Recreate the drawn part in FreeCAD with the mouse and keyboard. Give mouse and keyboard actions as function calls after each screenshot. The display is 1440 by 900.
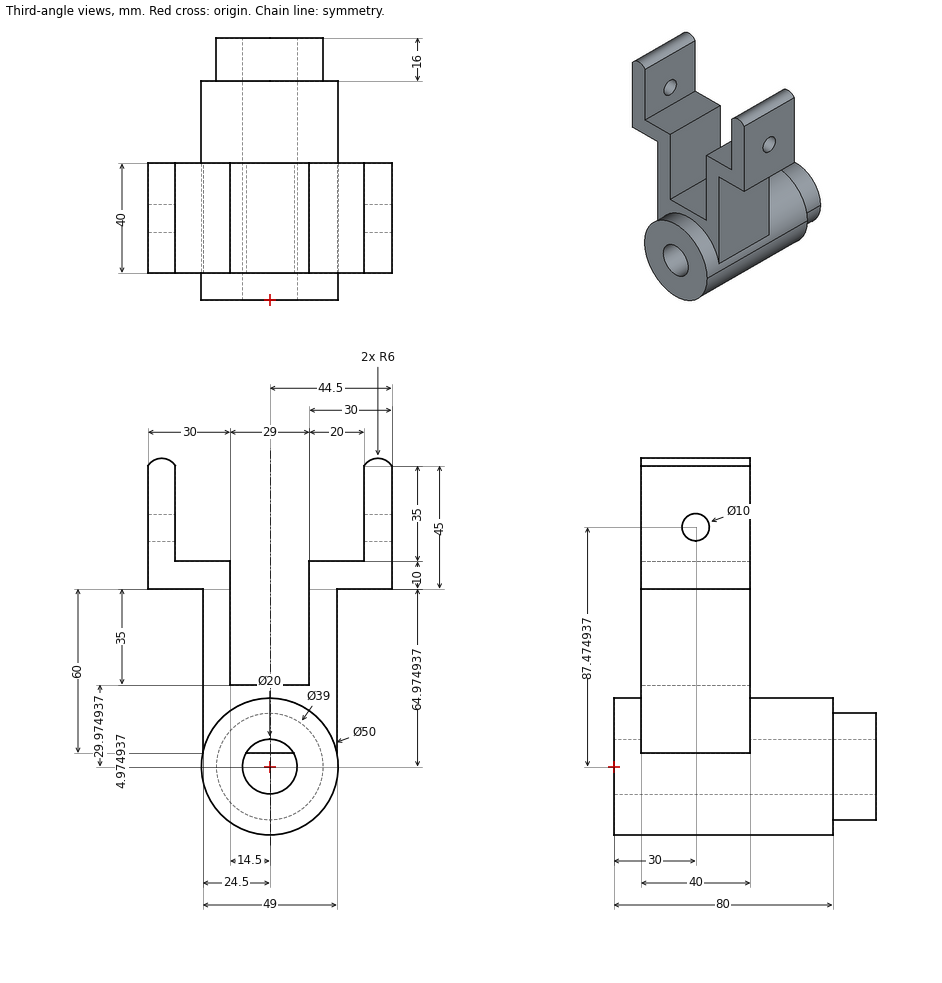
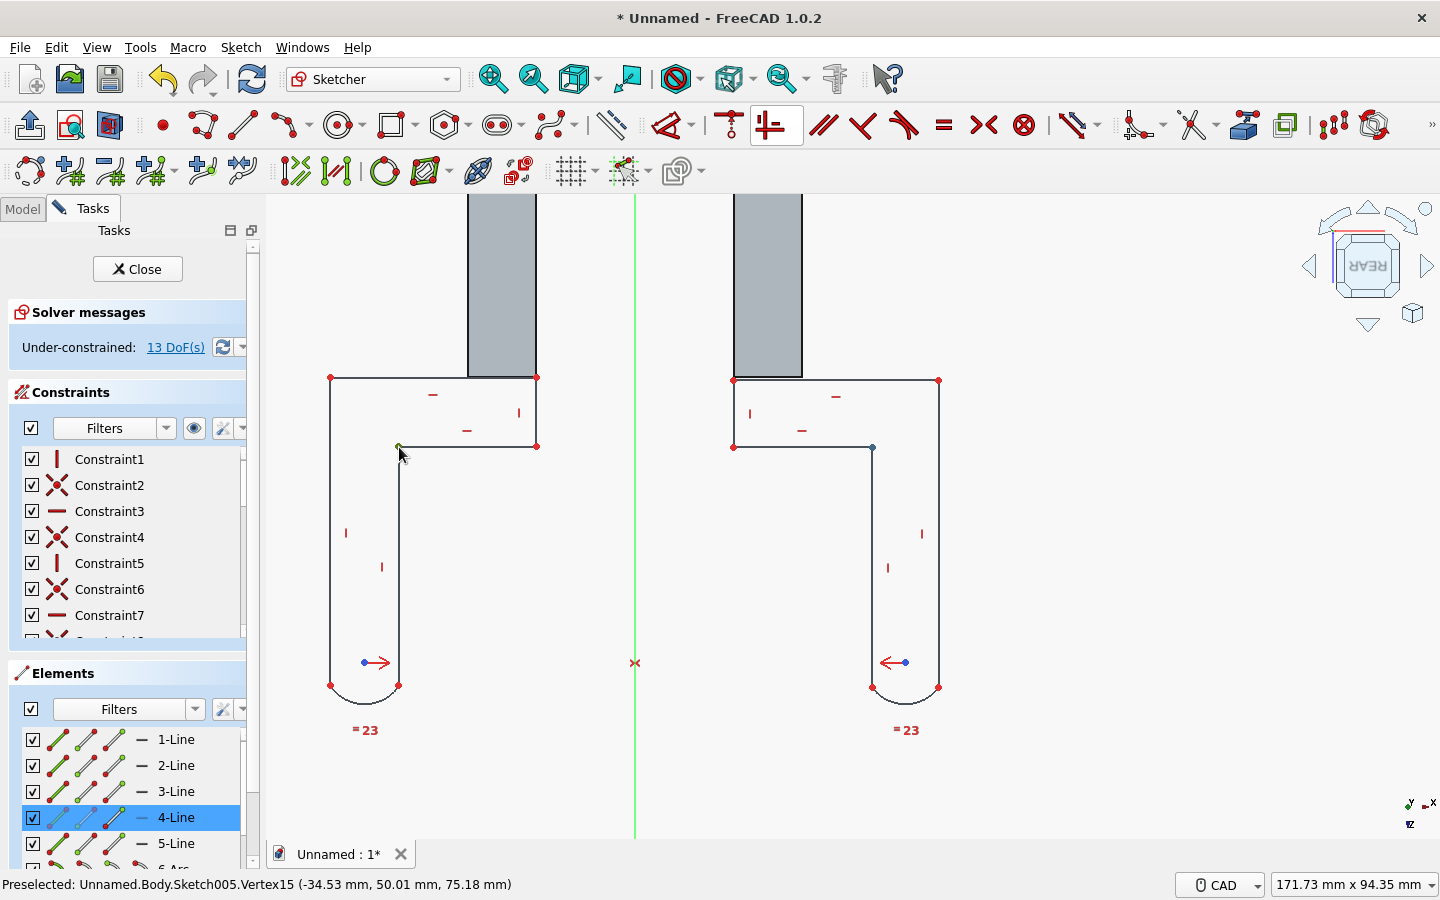
click(635, 769)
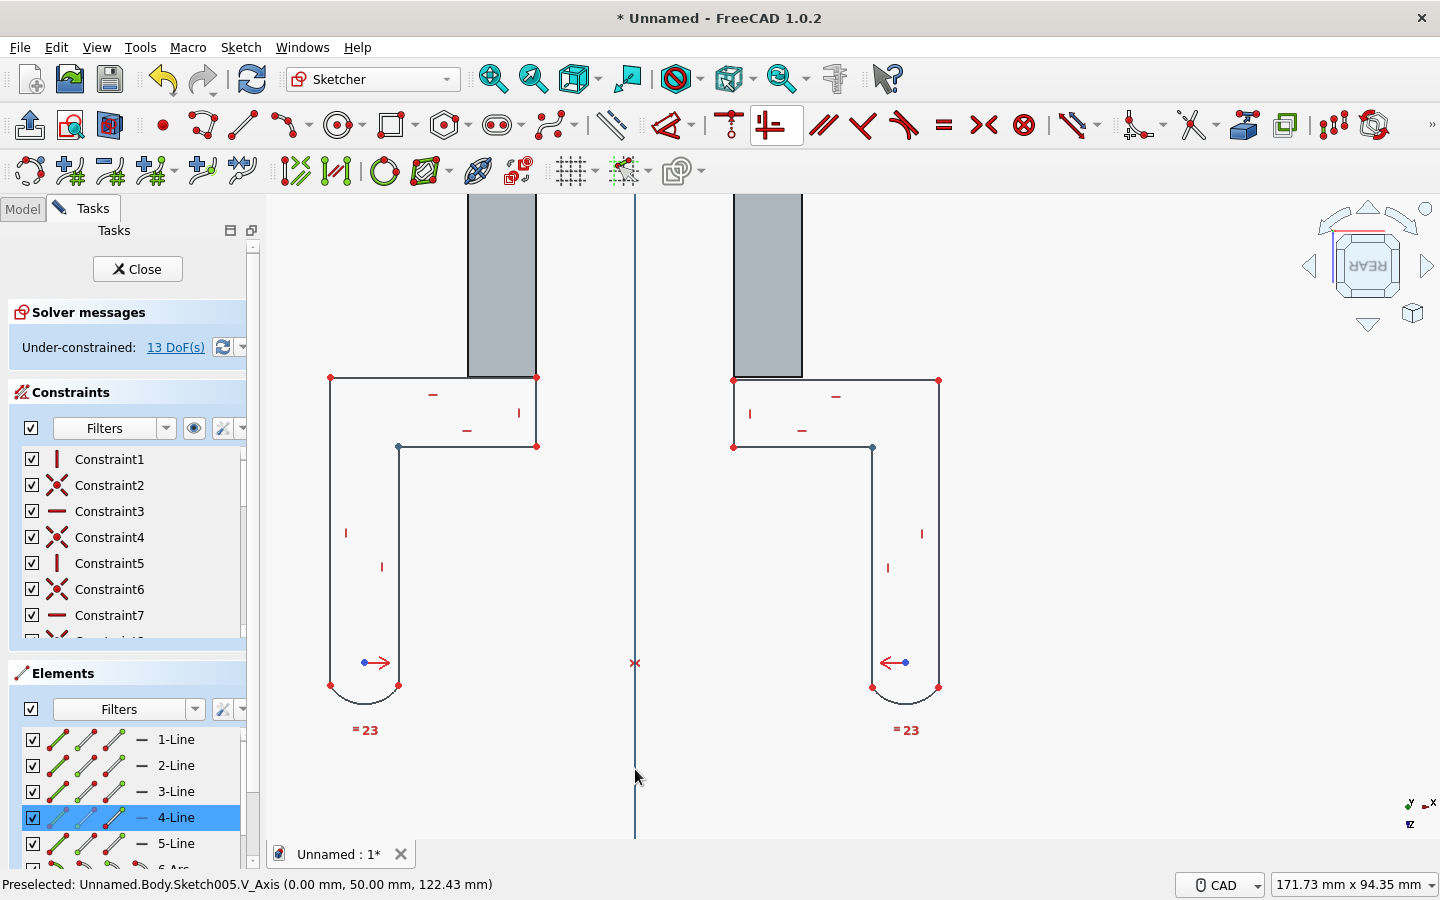
click(984, 126)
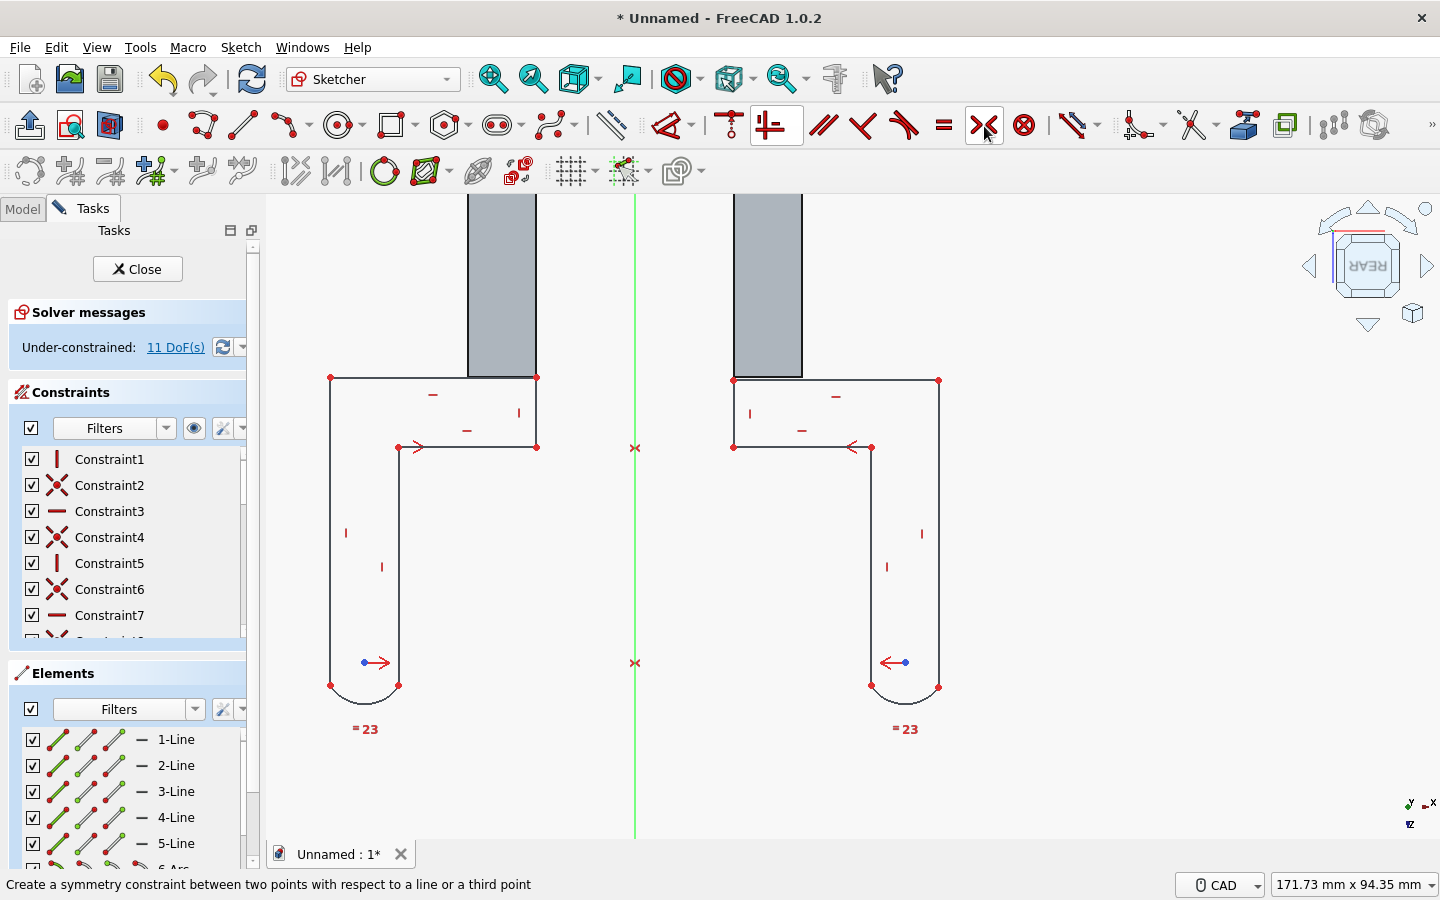
click(734, 380)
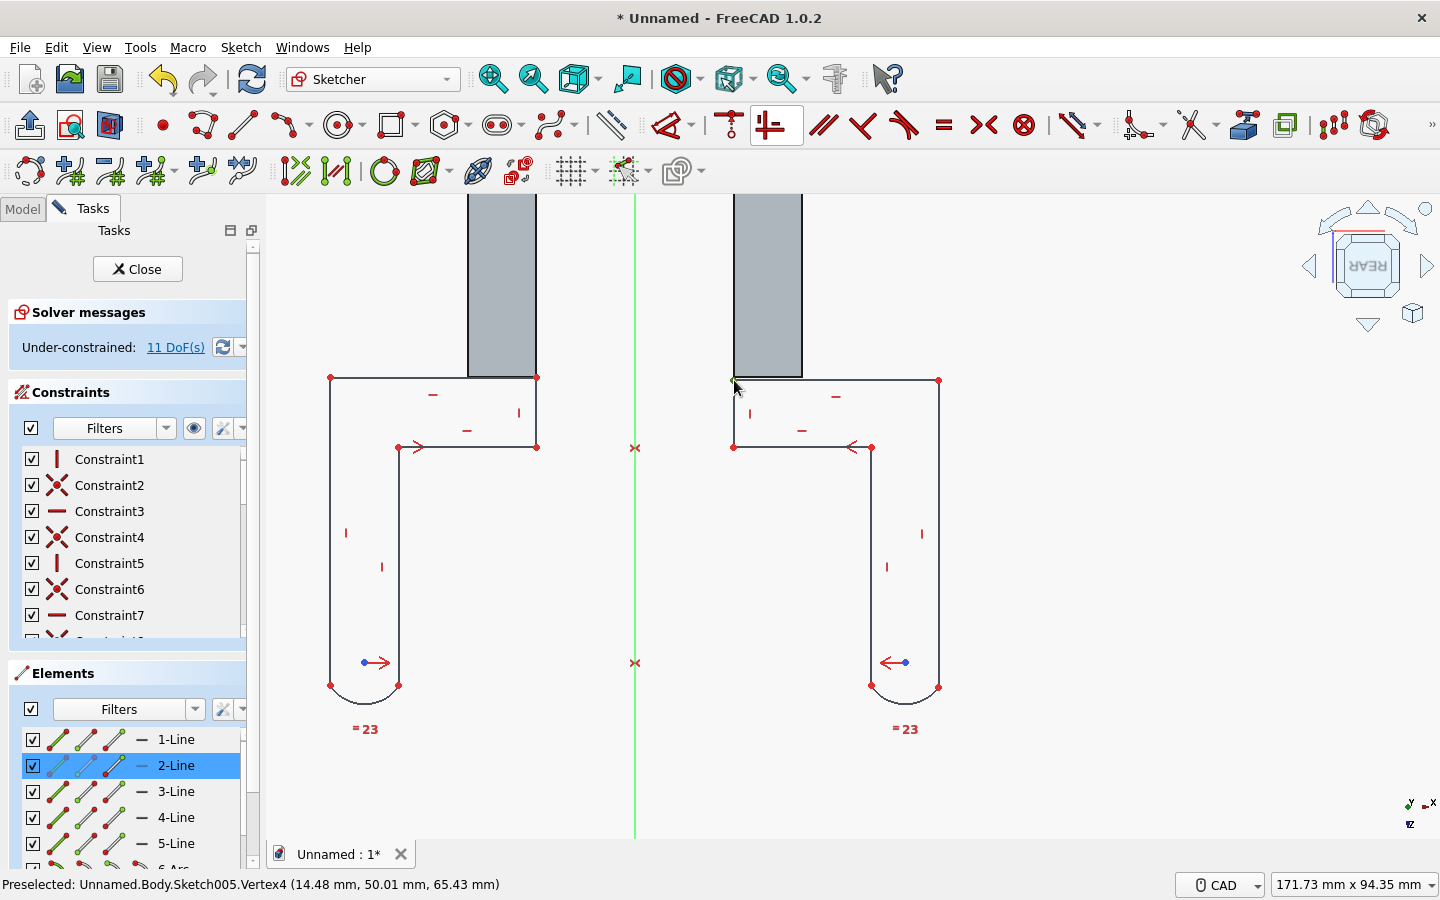
click(536, 378)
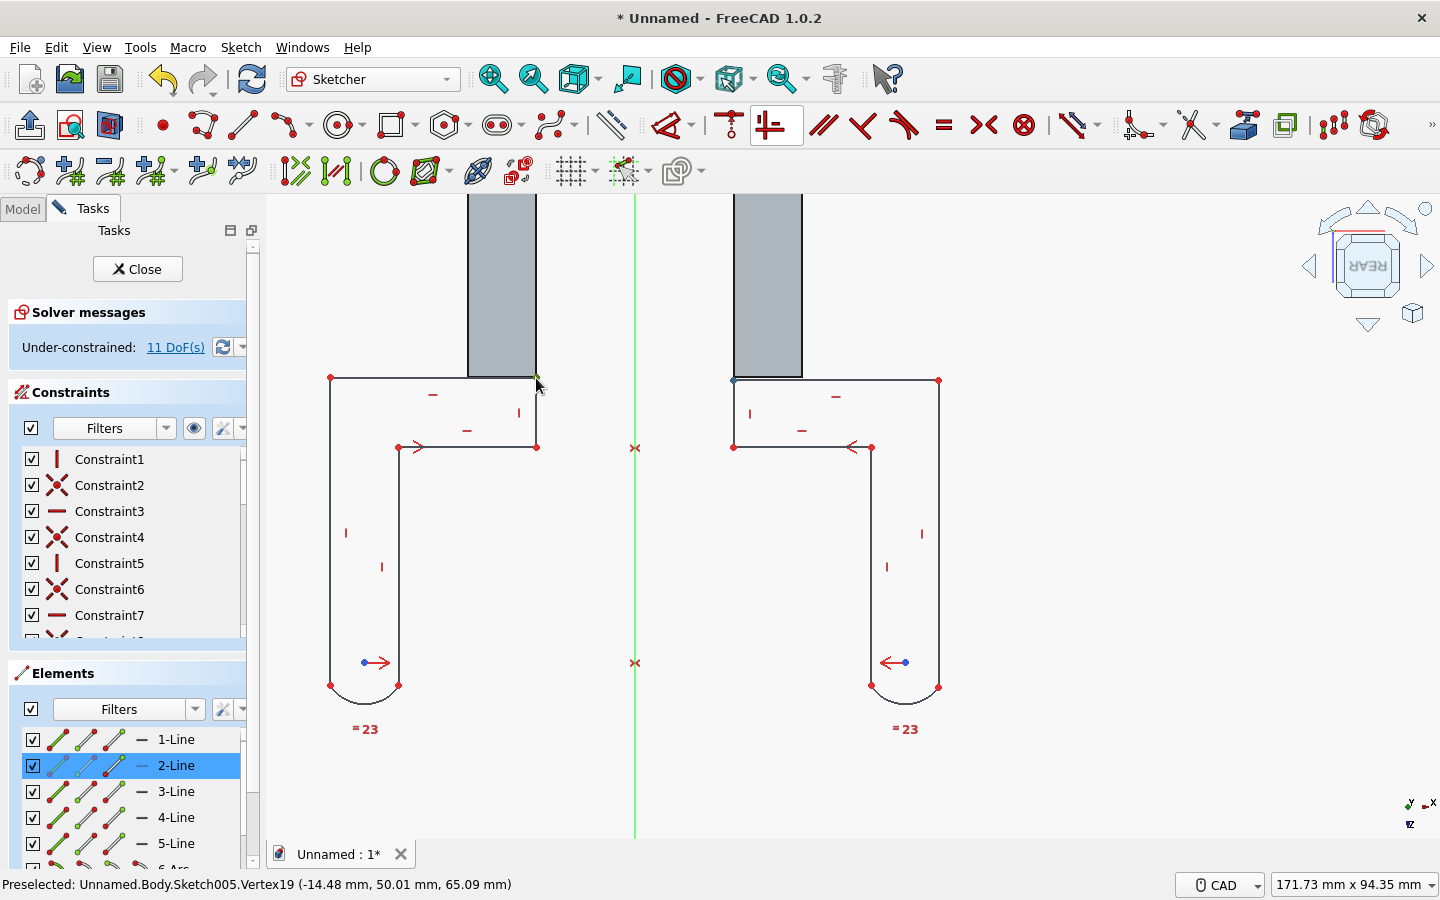
click(635, 769)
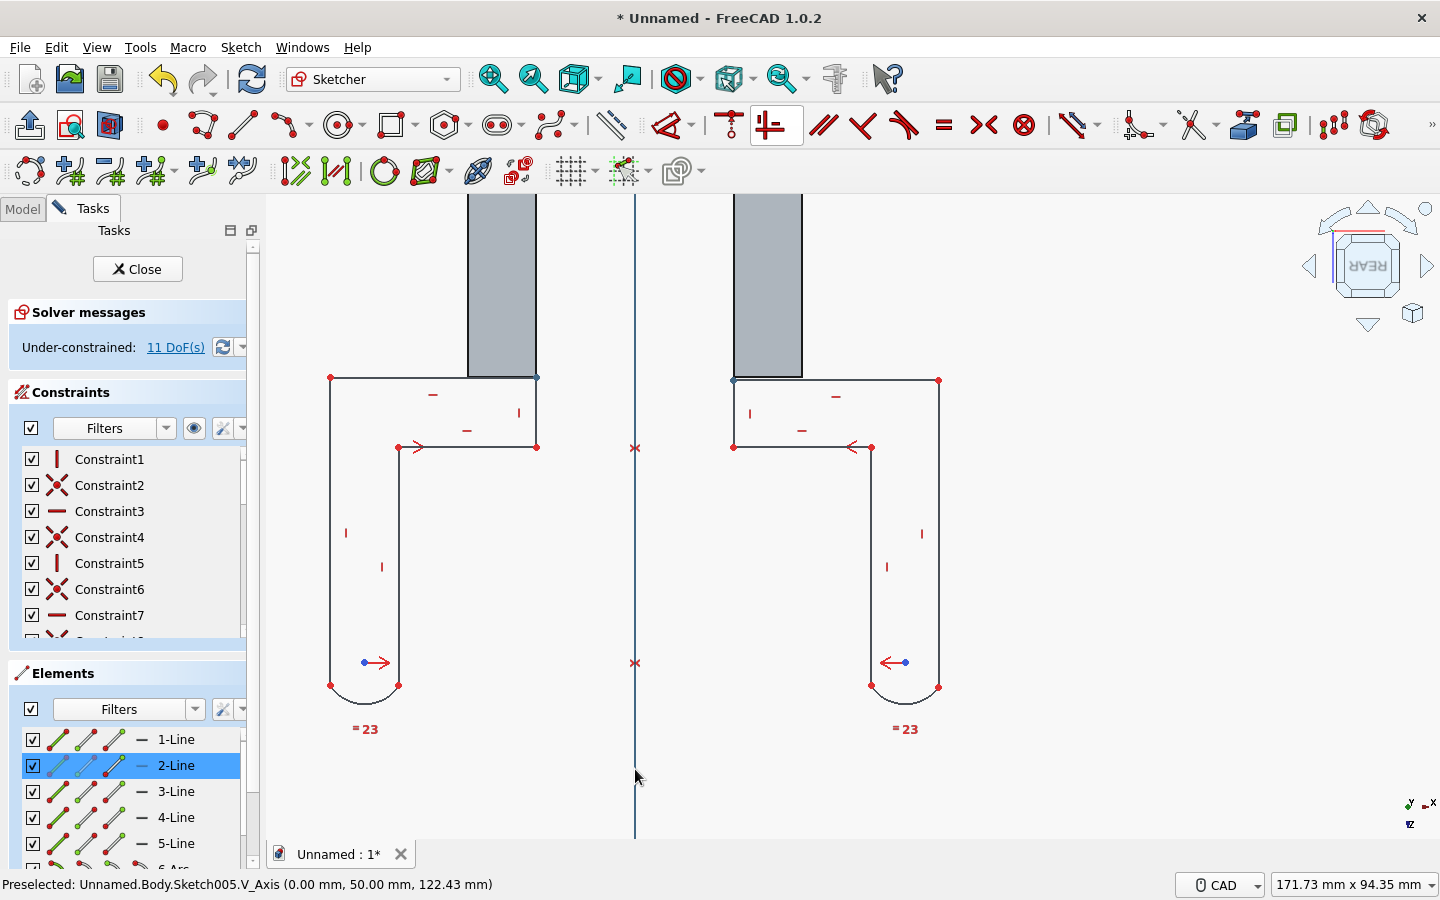
key(s)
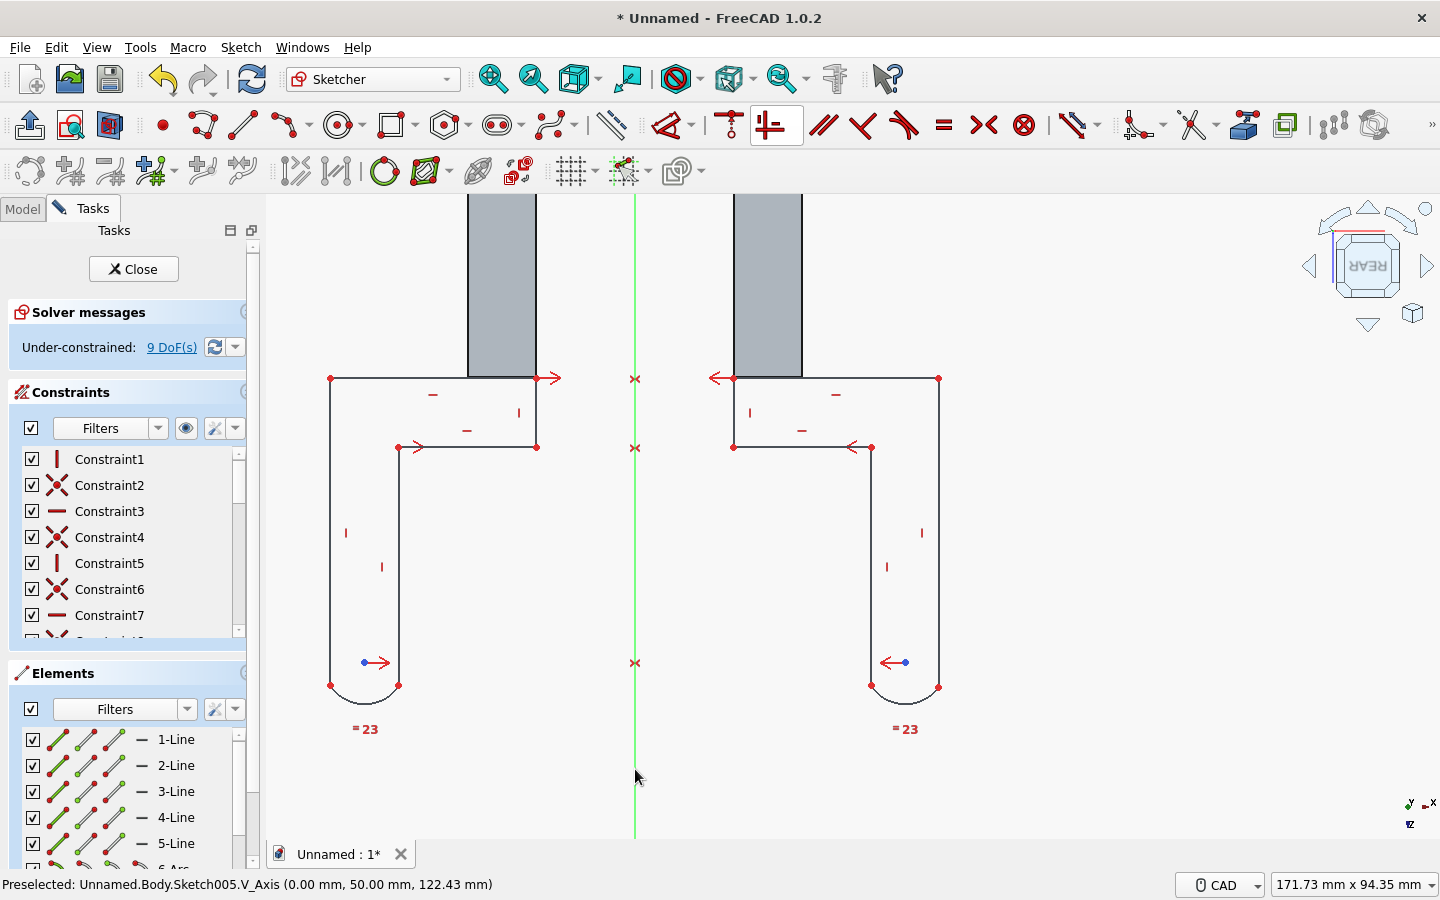
click(666, 126)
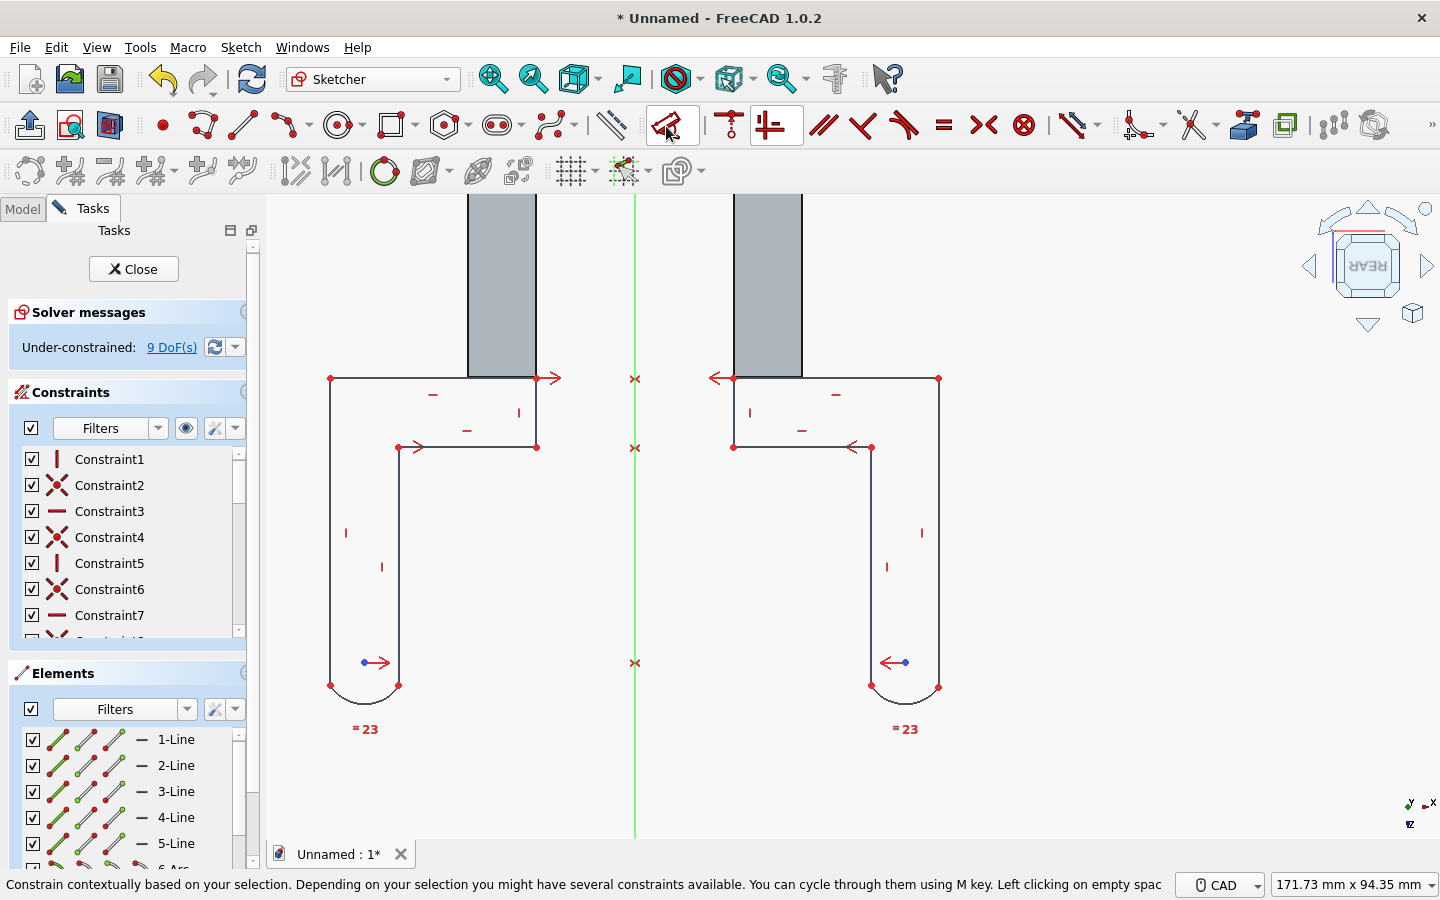
click(889, 701)
click(876, 730)